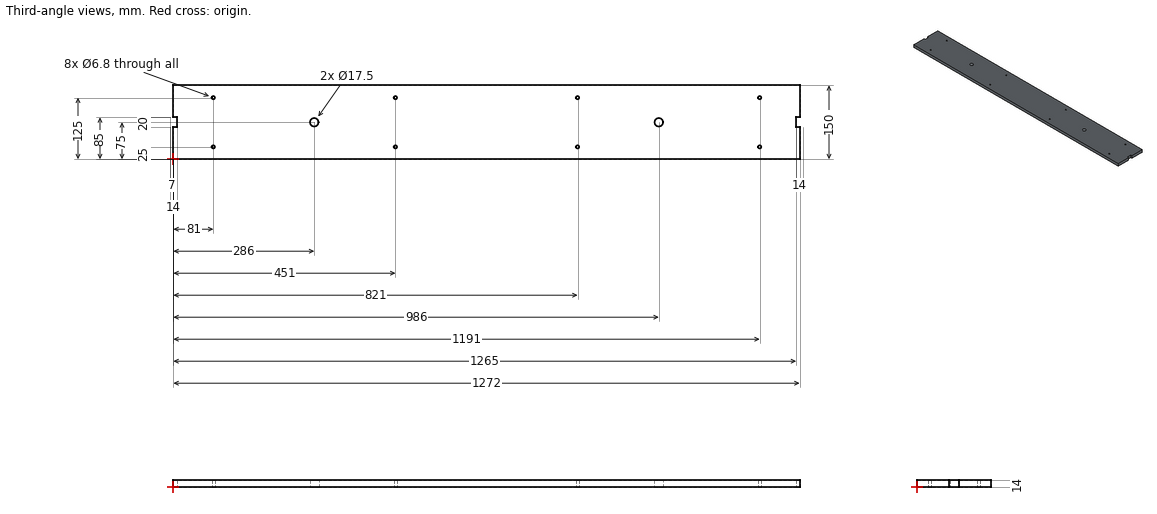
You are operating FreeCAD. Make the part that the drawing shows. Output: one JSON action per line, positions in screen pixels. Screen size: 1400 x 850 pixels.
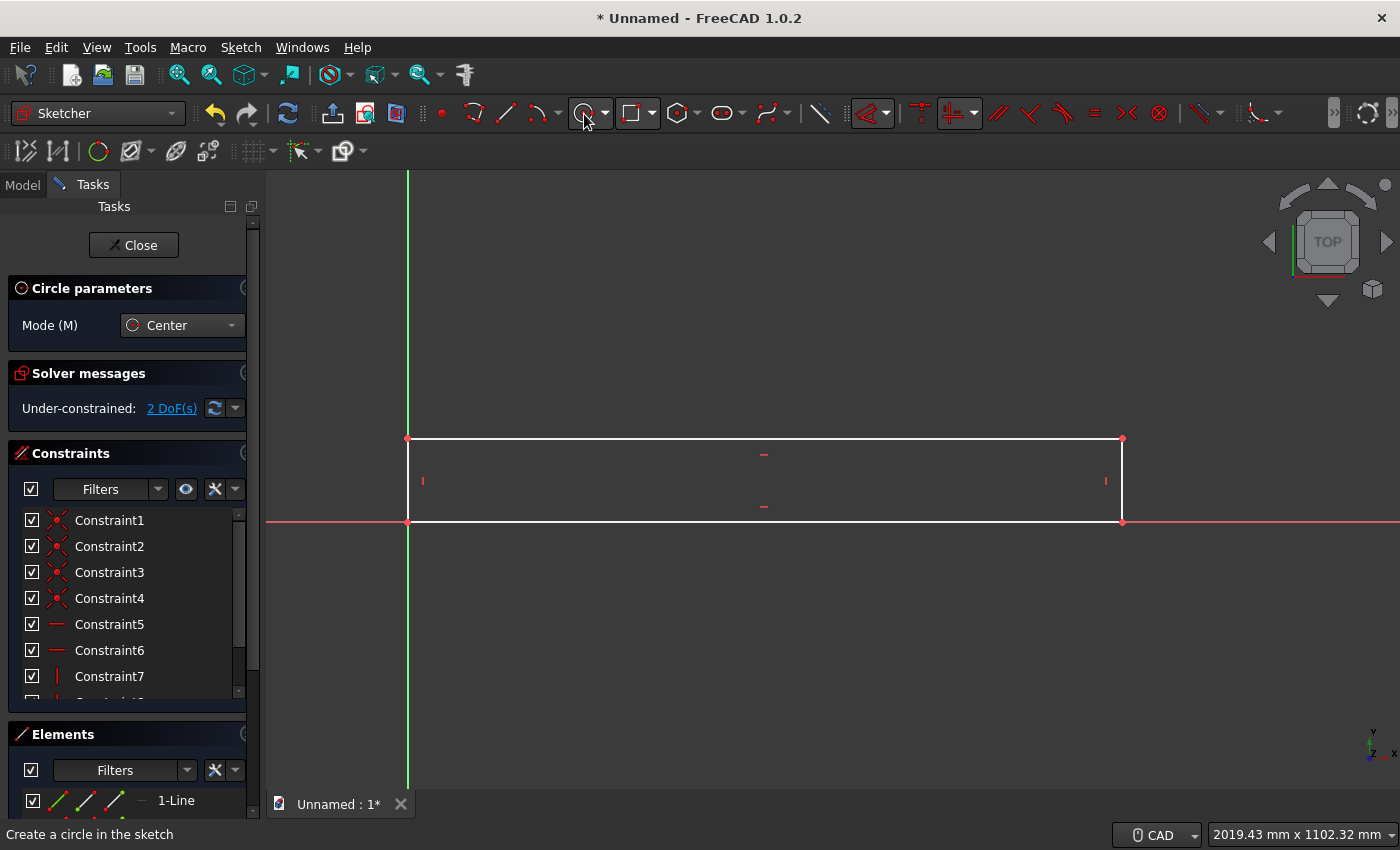
{"action": "scroll", "coordinate": [568, 480], "scroll_direction": "up", "scroll_amount": 8}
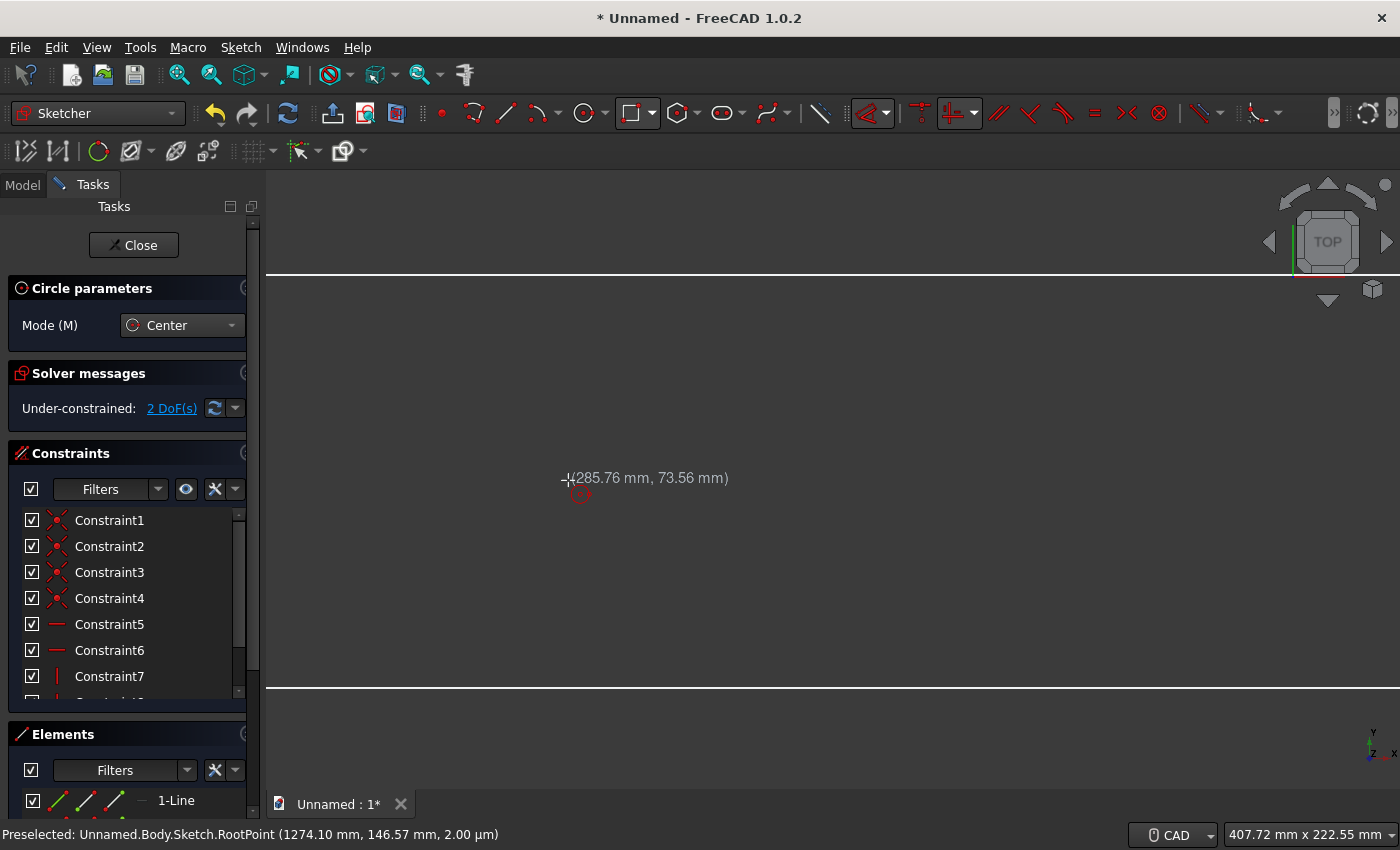
{"action": "scroll", "coordinate": [568, 480], "scroll_direction": "down", "scroll_amount": 8}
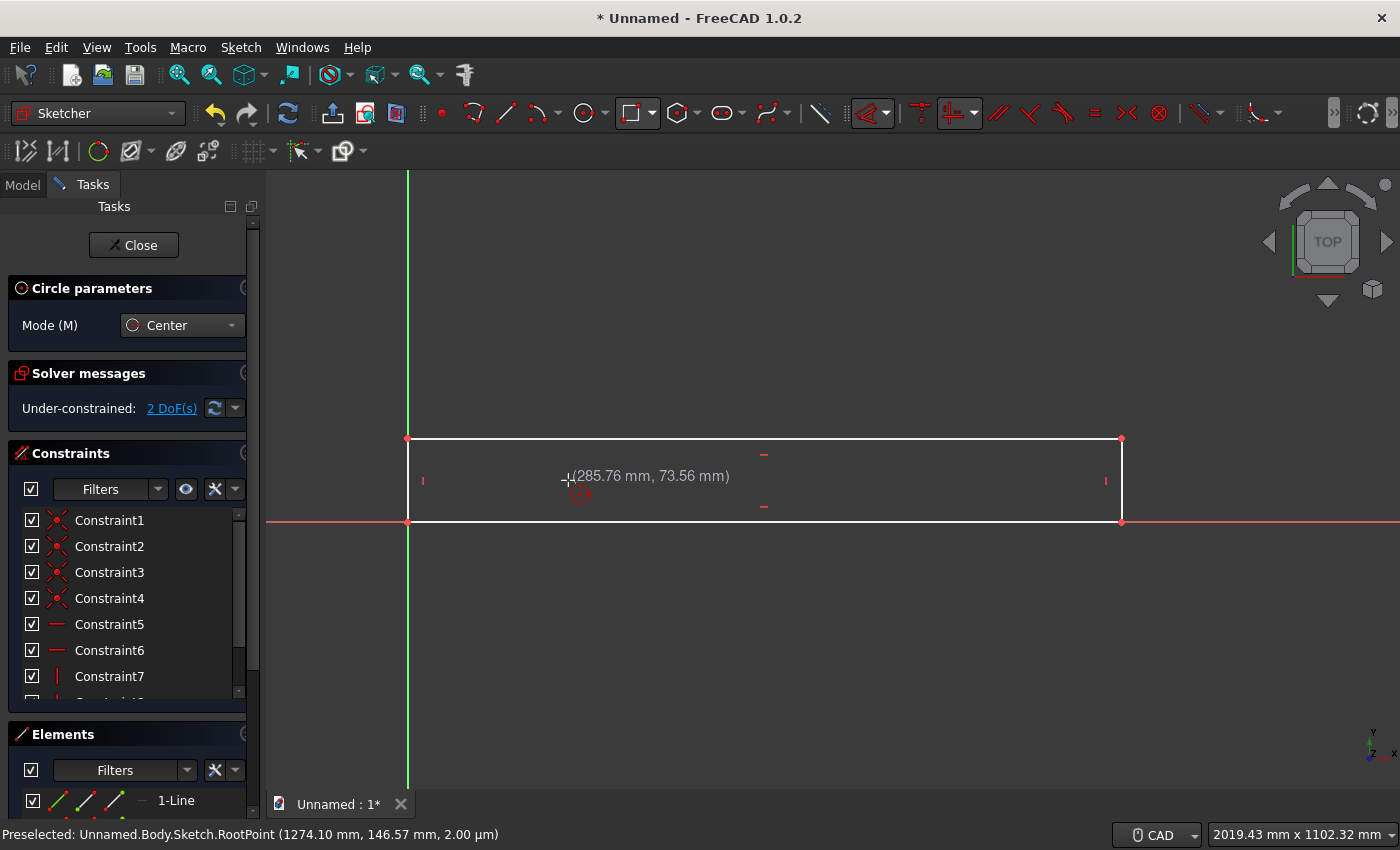
{"action": "left_click", "coordinate": [568, 480]}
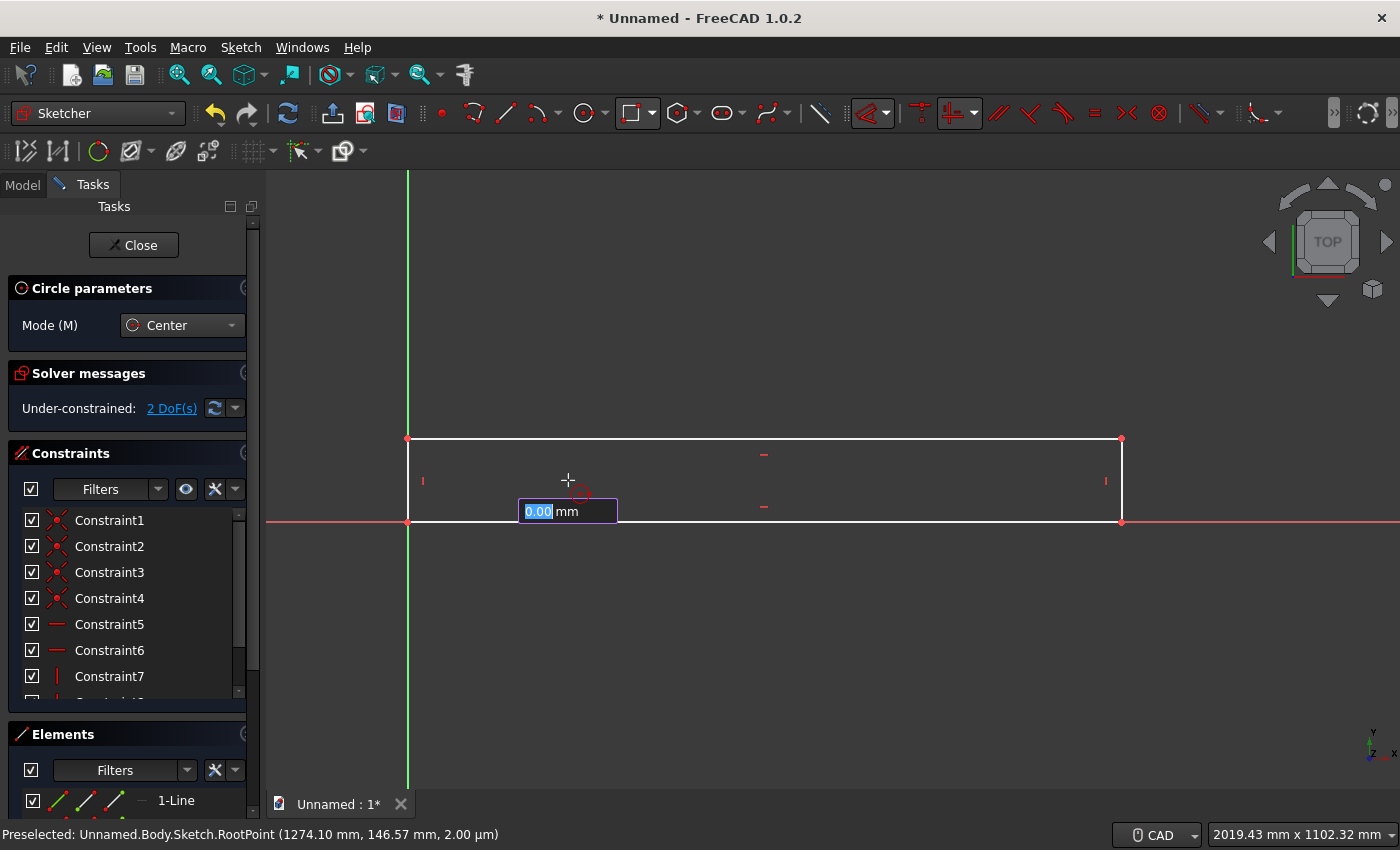
{"action": "scroll", "coordinate": [572, 477], "scroll_direction": "up", "scroll_amount": 6}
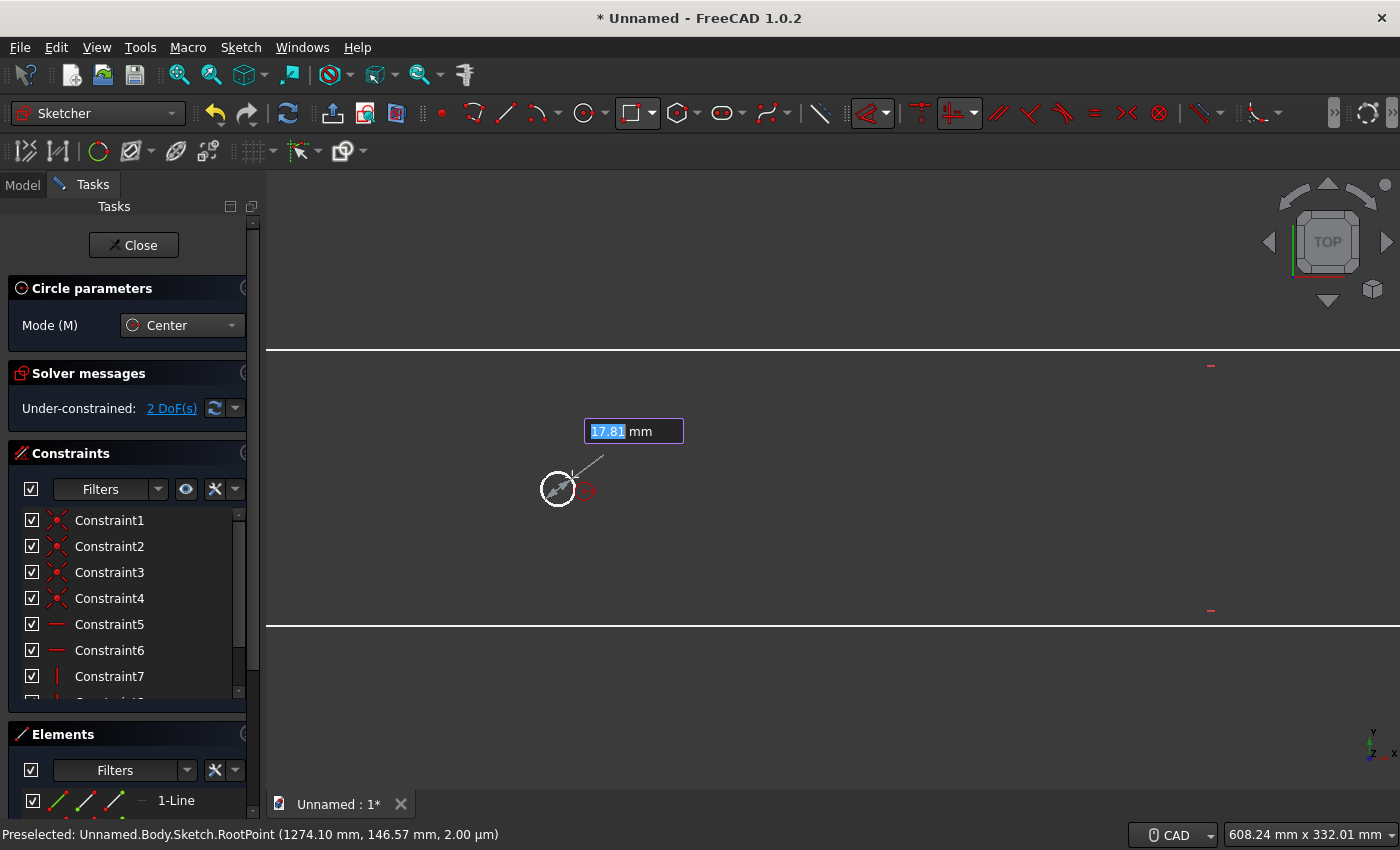
{"action": "left_click", "coordinate": [570, 475]}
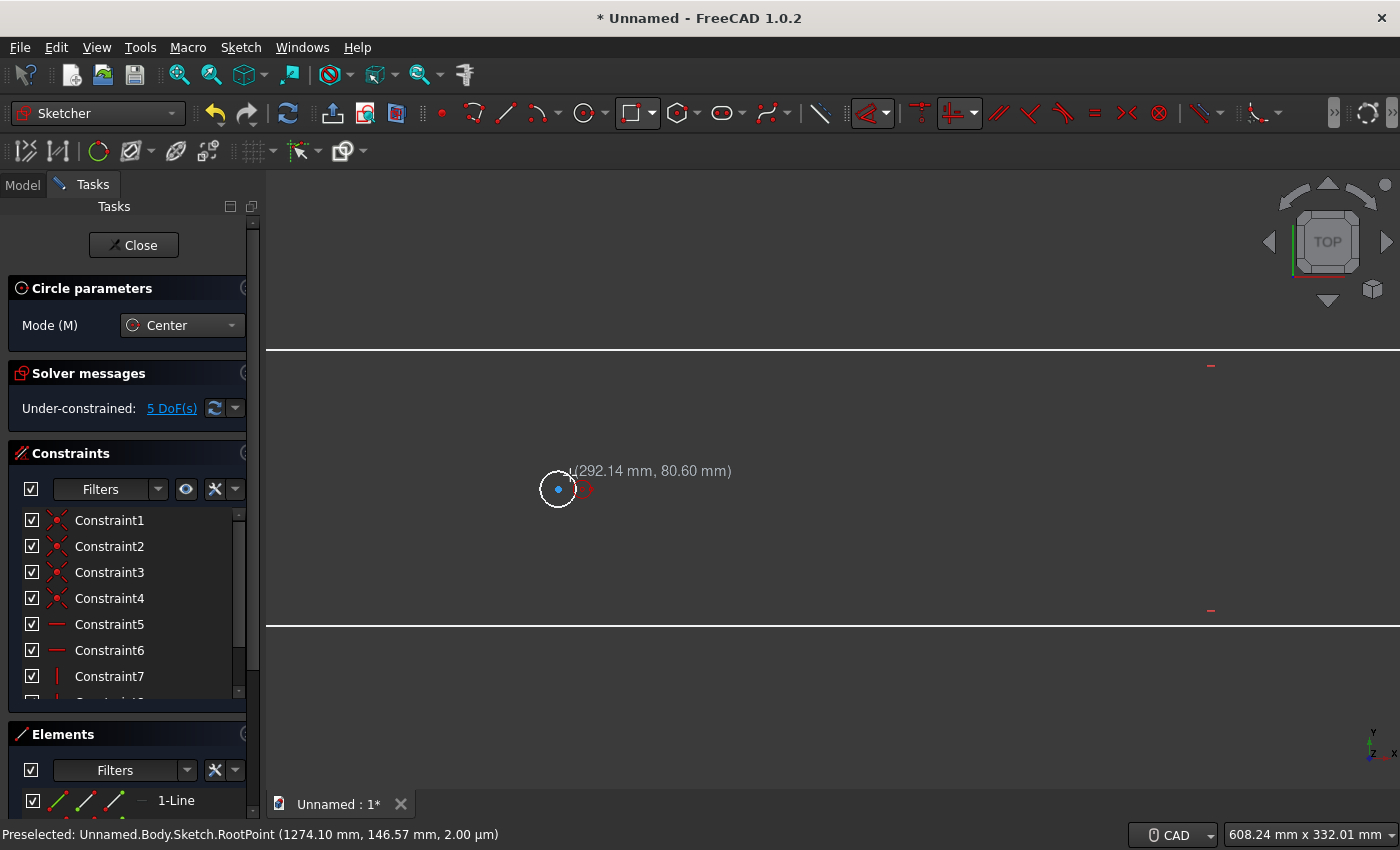
{"action": "scroll", "coordinate": [572, 477], "scroll_direction": "down", "scroll_amount": 6}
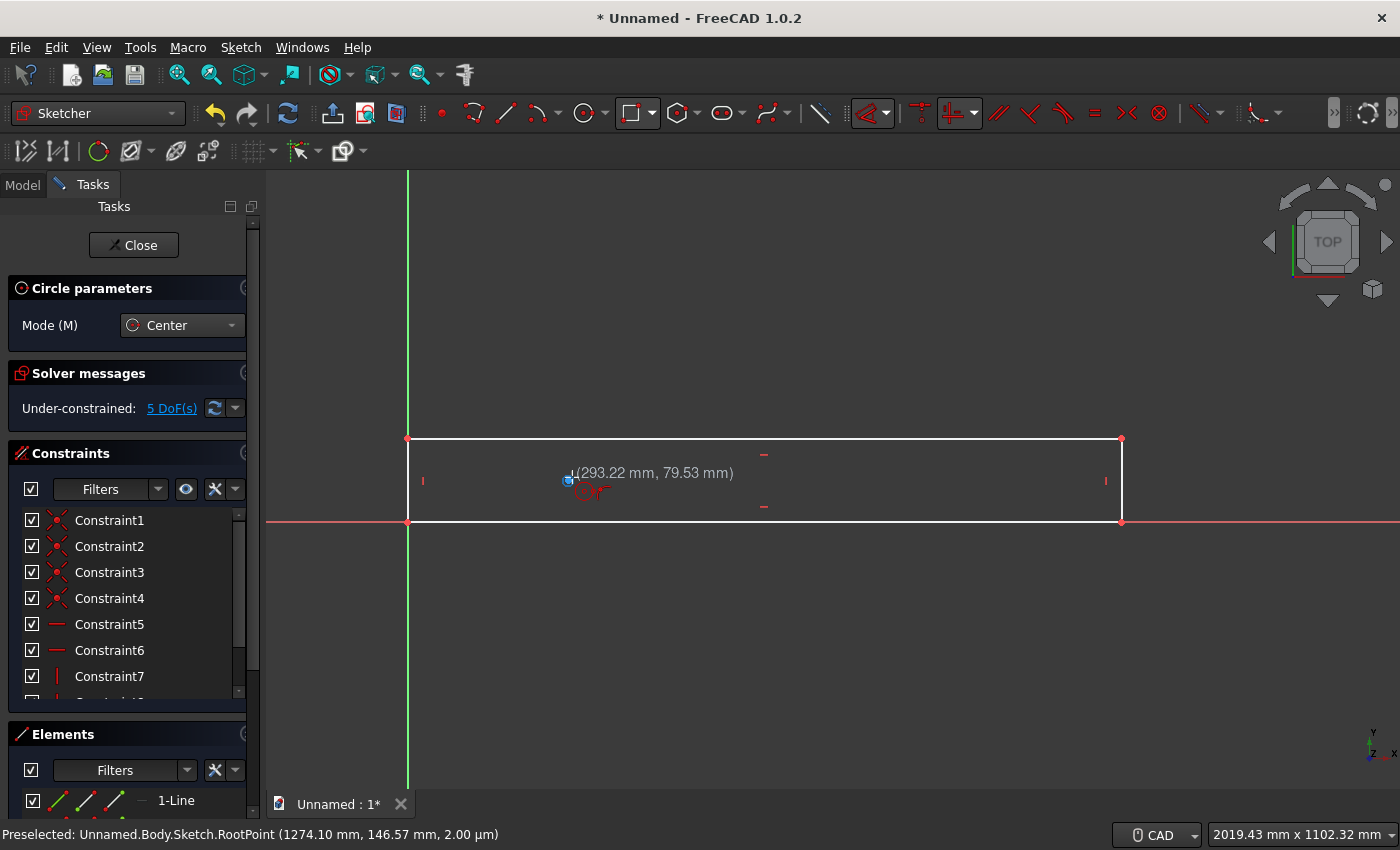
{"action": "scroll", "coordinate": [961, 480], "scroll_direction": "up", "scroll_amount": 8}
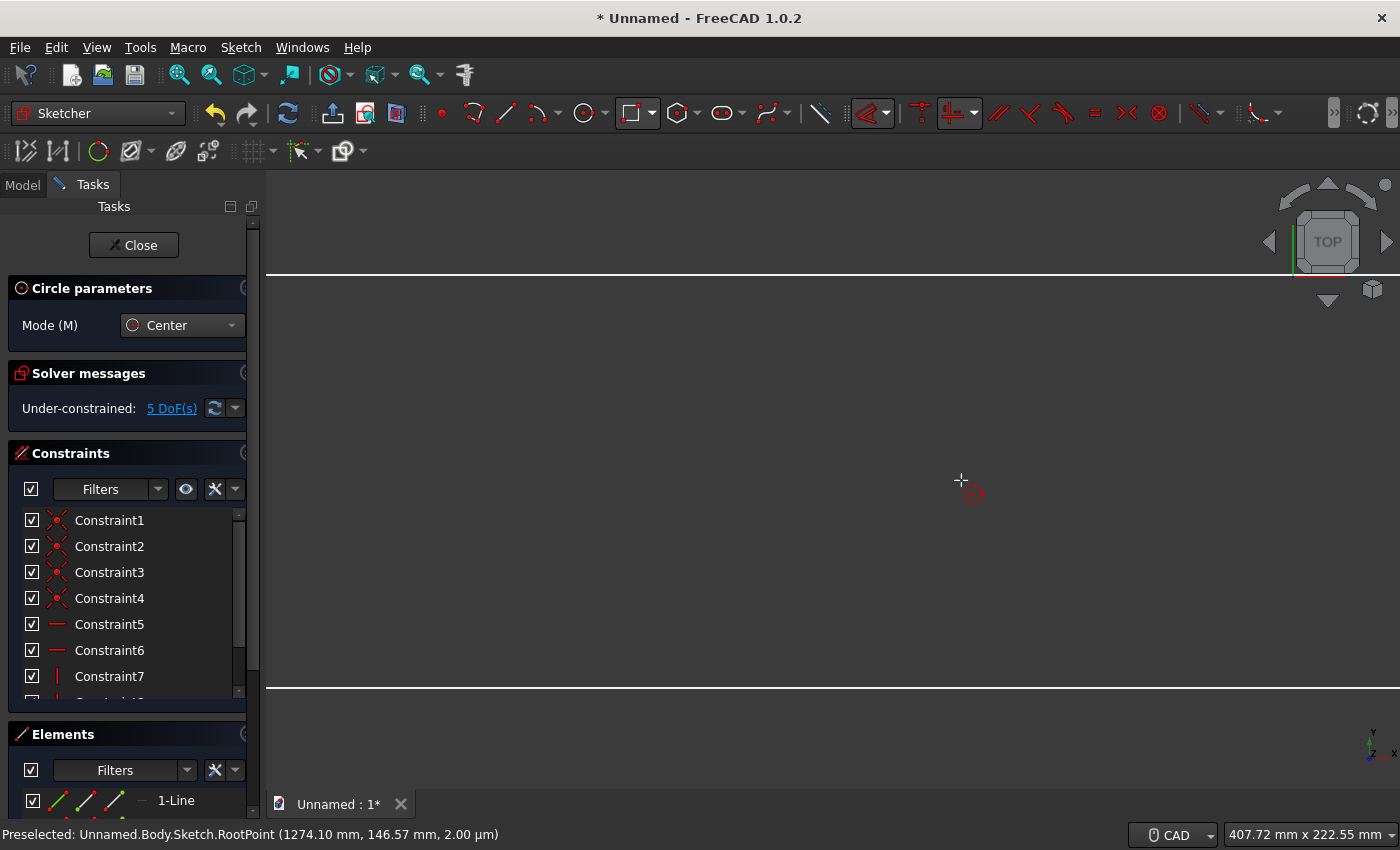
{"action": "scroll", "coordinate": [961, 480], "scroll_direction": "down", "scroll_amount": 8}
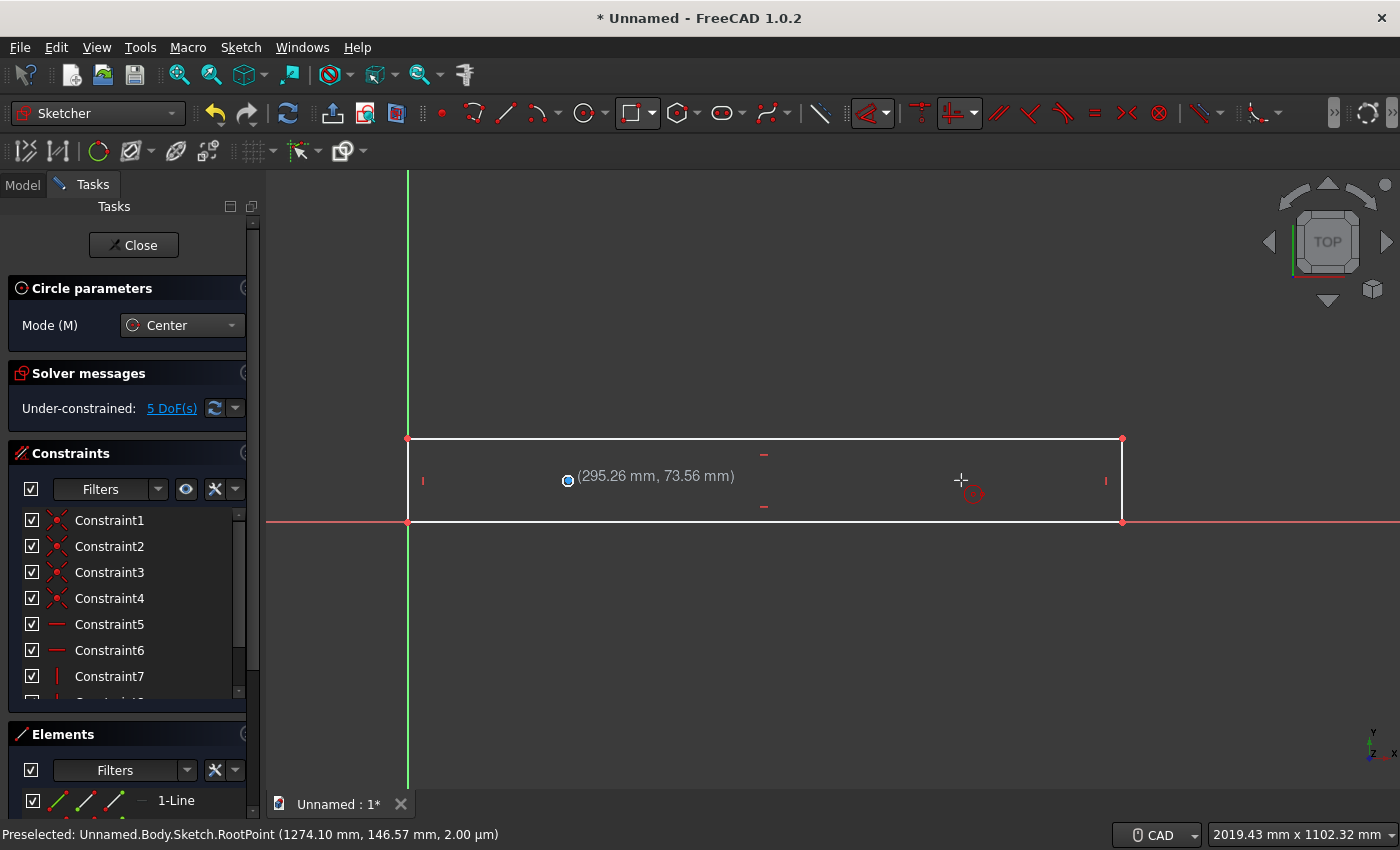
{"action": "left_click", "coordinate": [961, 480]}